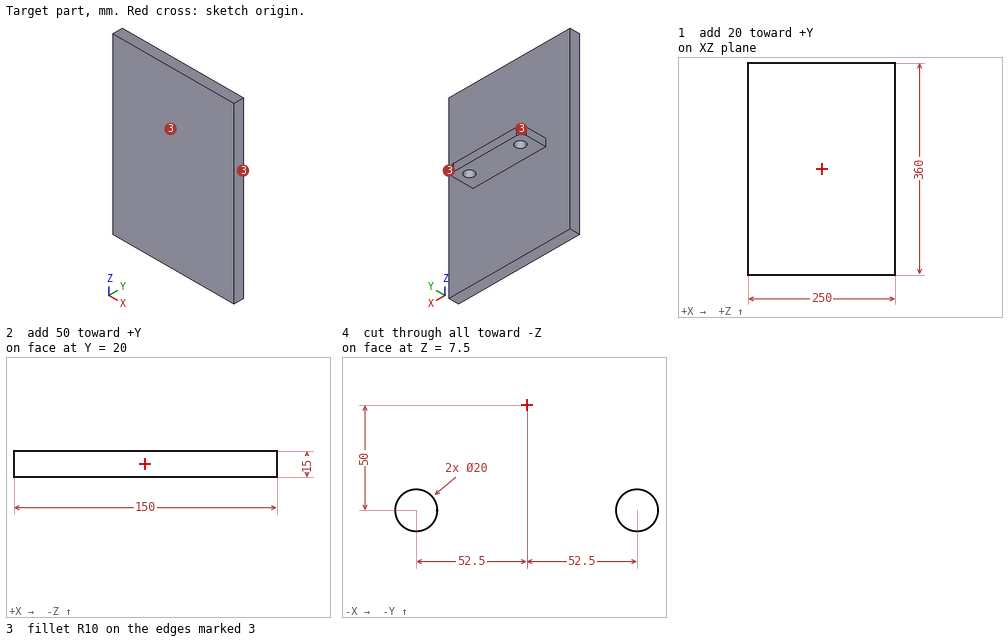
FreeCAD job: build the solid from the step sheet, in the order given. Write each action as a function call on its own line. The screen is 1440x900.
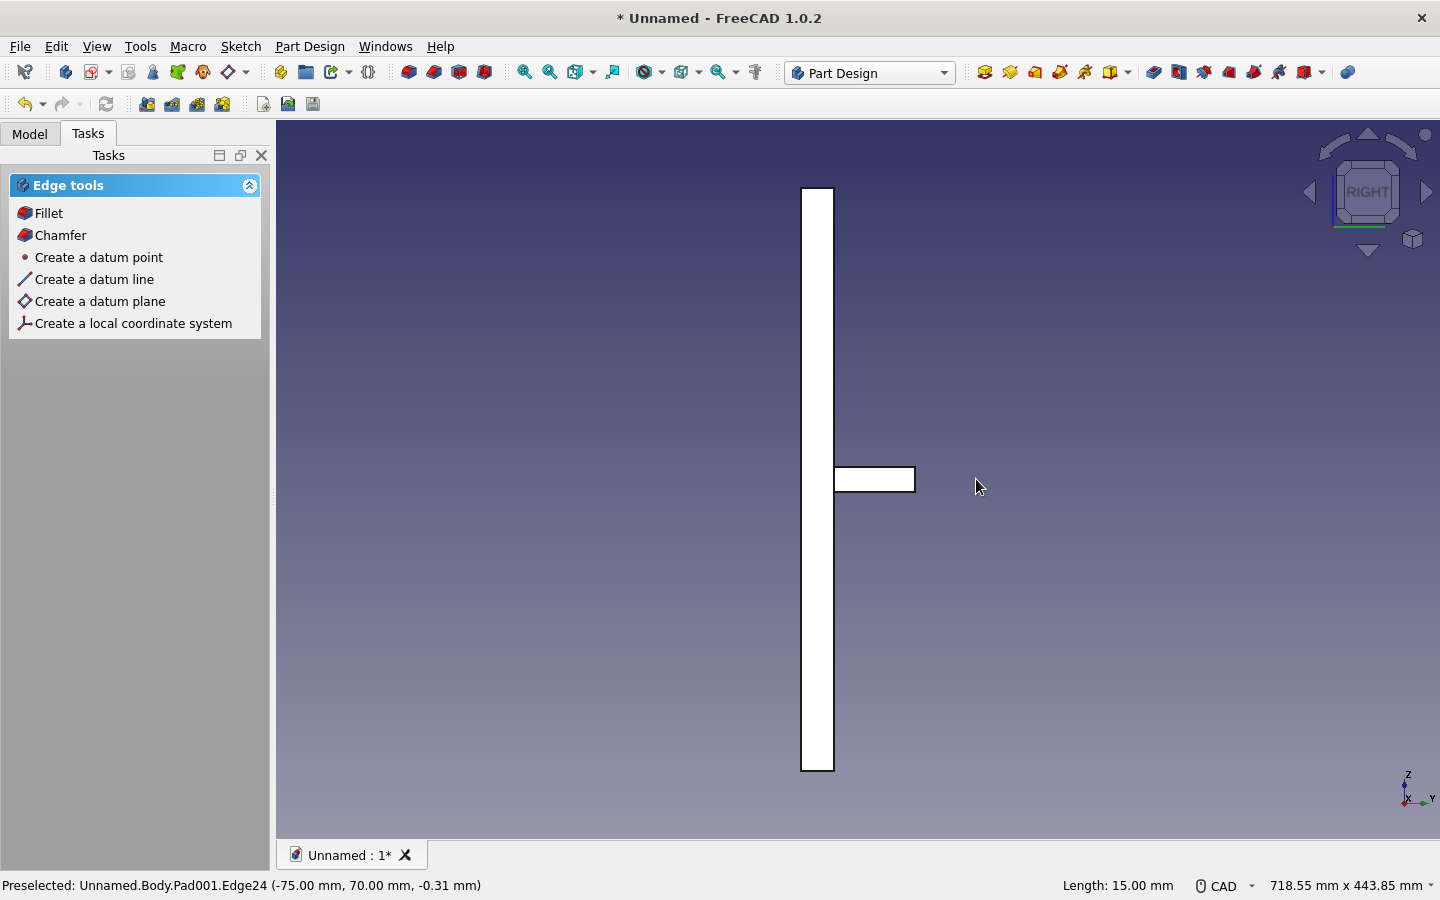
click(915, 479, ctrl)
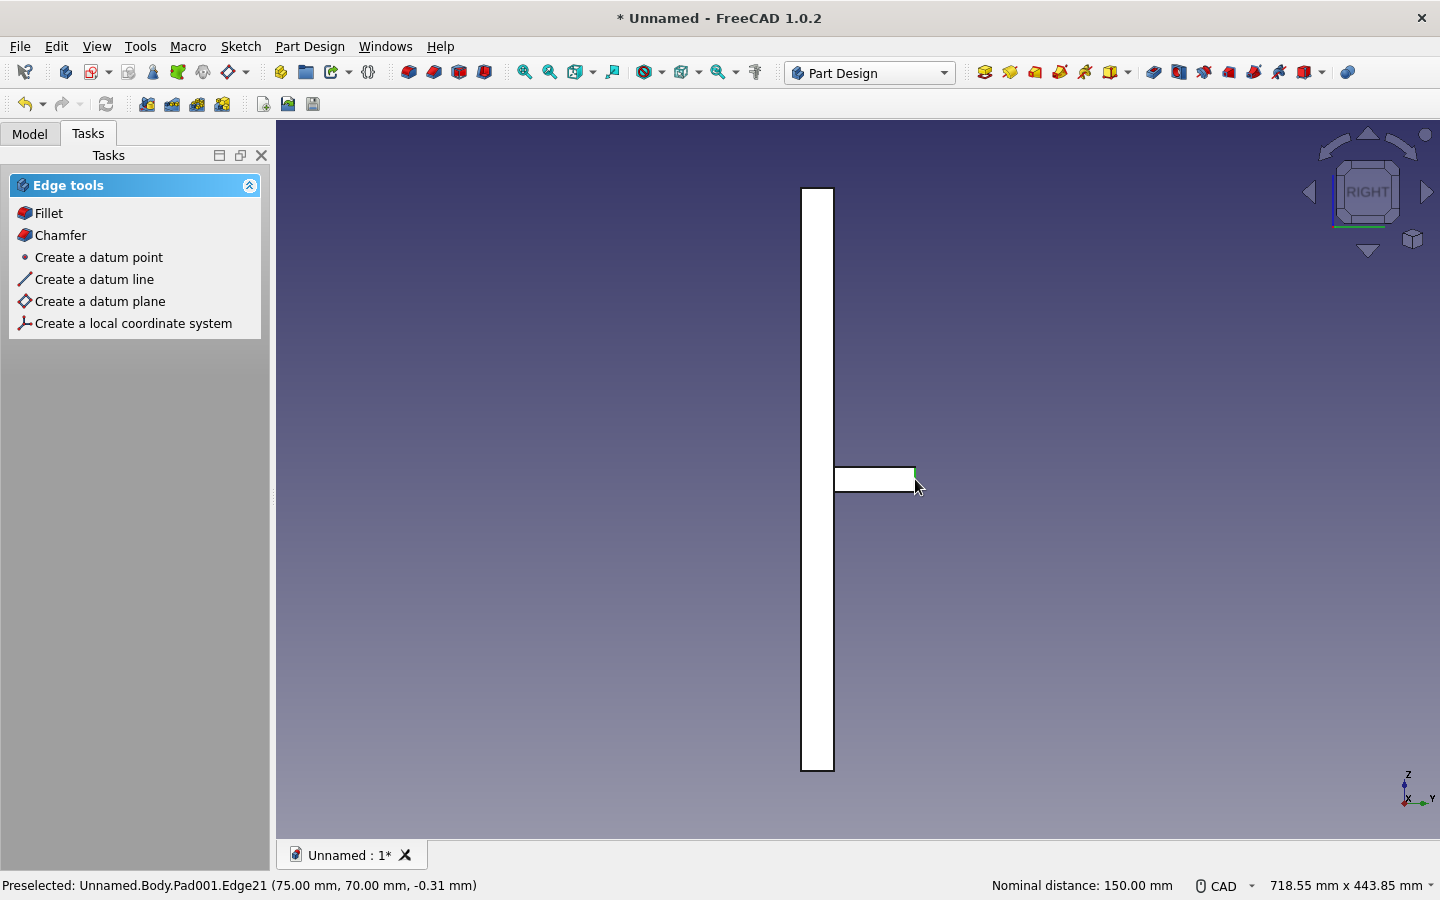
click(409, 72)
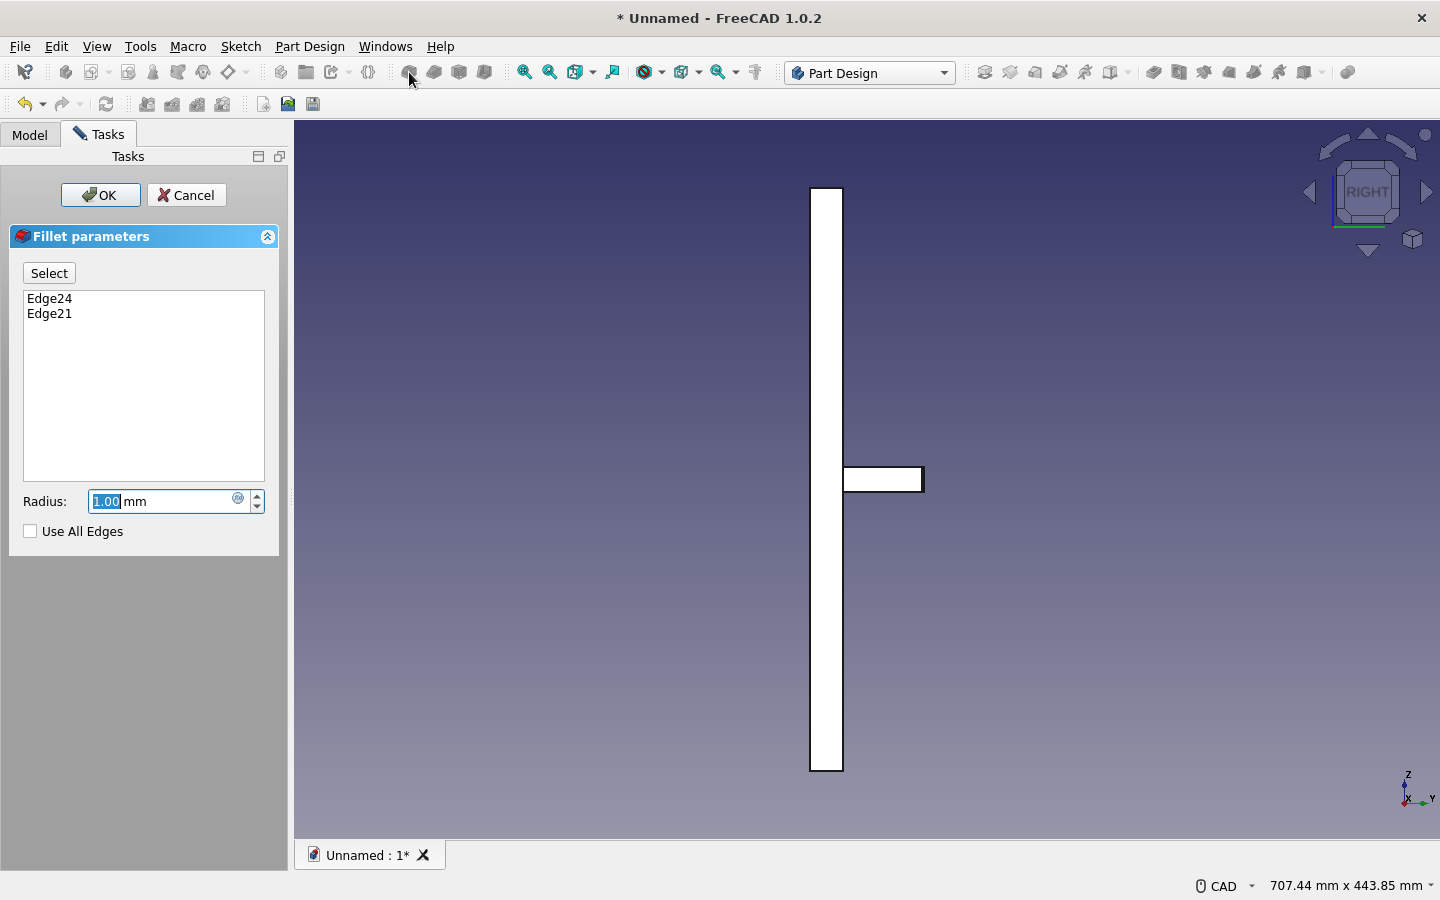
text(10)
key(Tab)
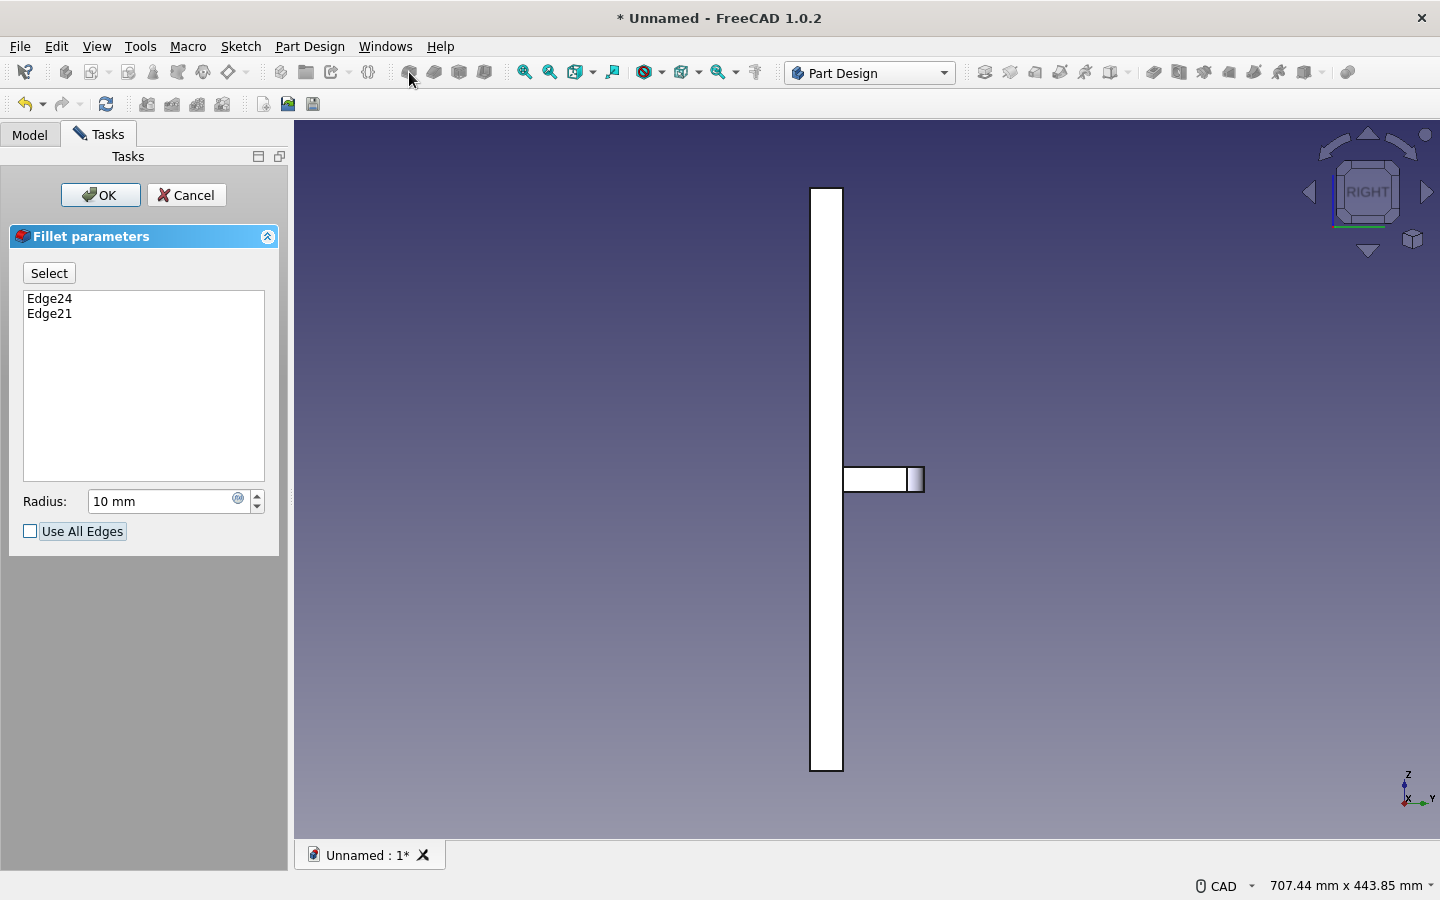
click(101, 195)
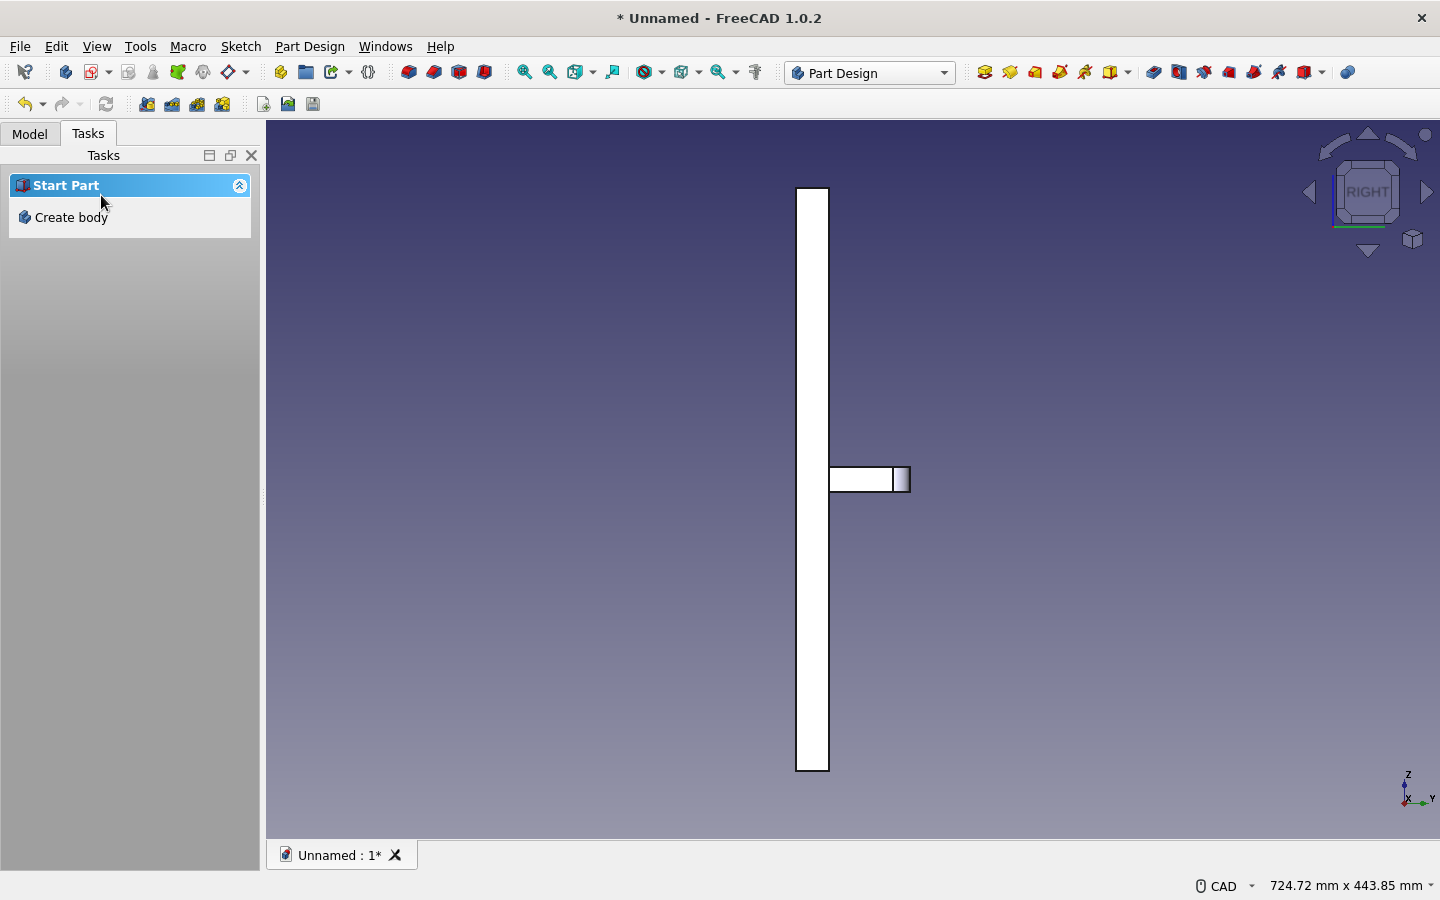
key(0)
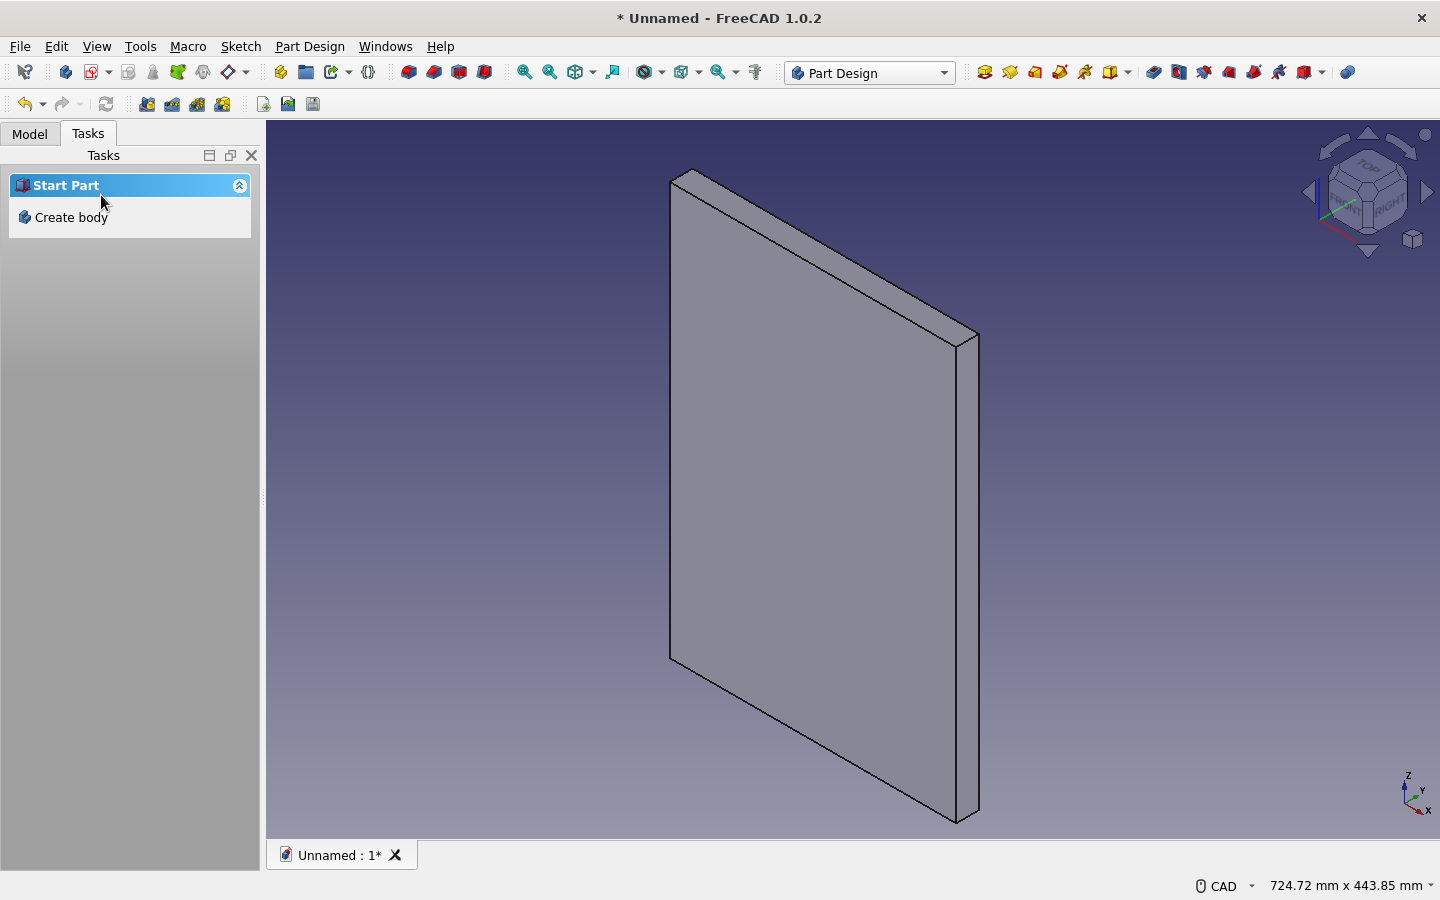
key(2)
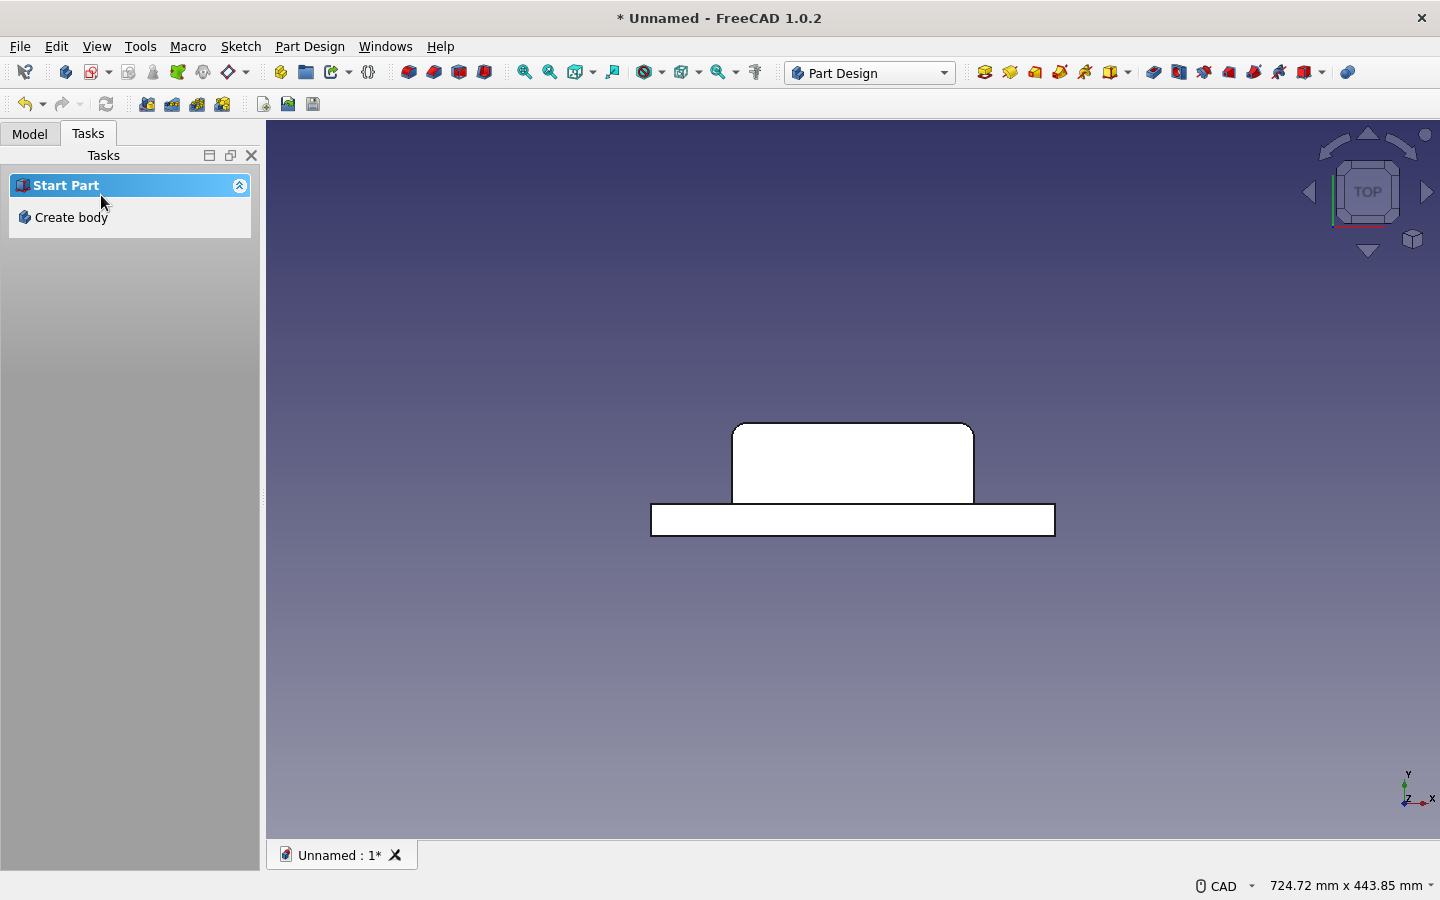
key(v)
key(f)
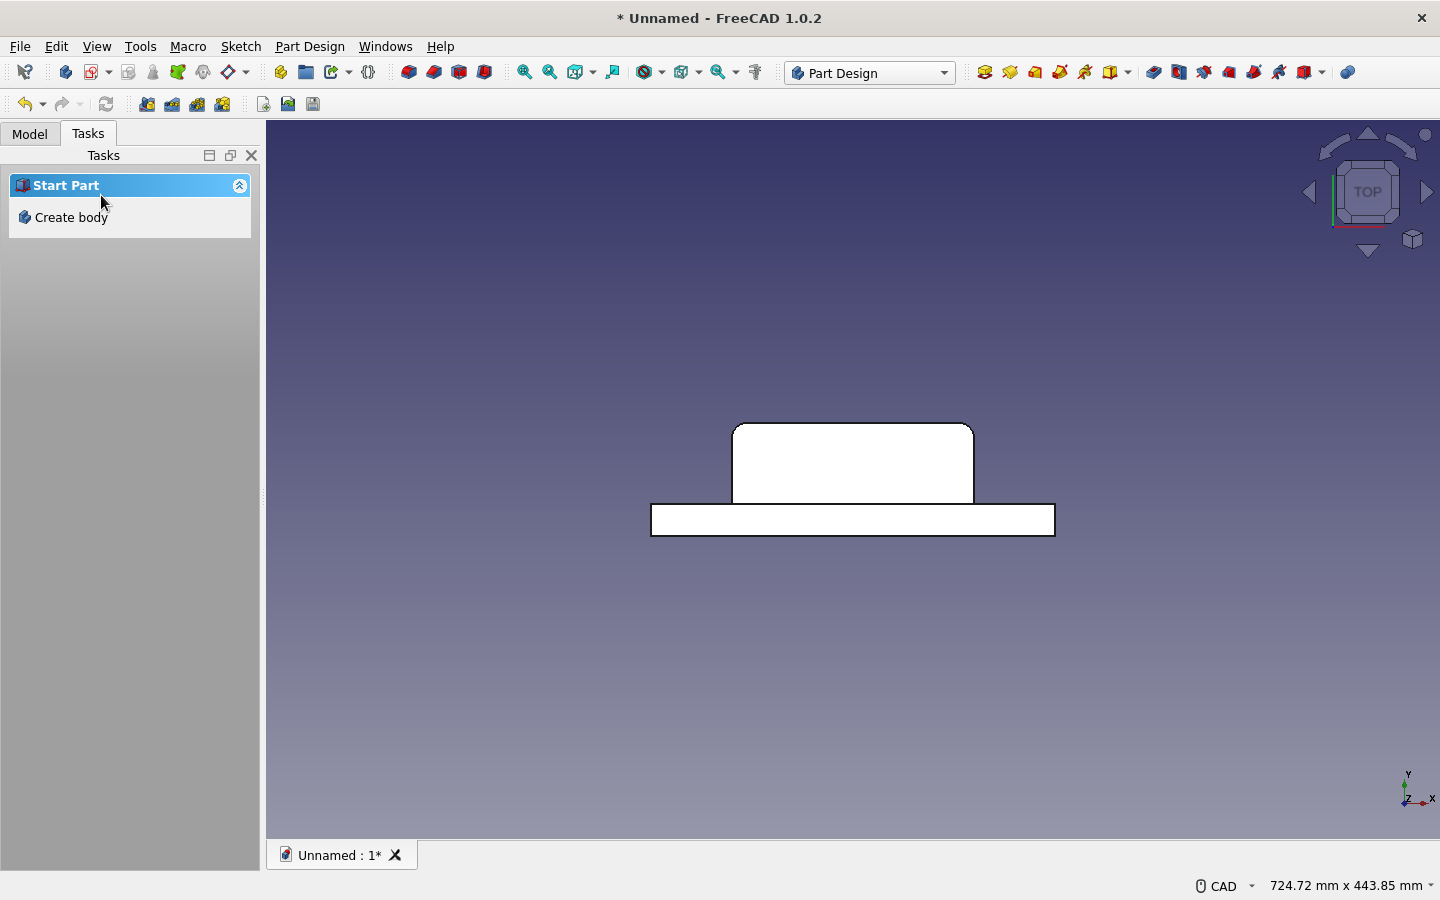
click(922, 462)